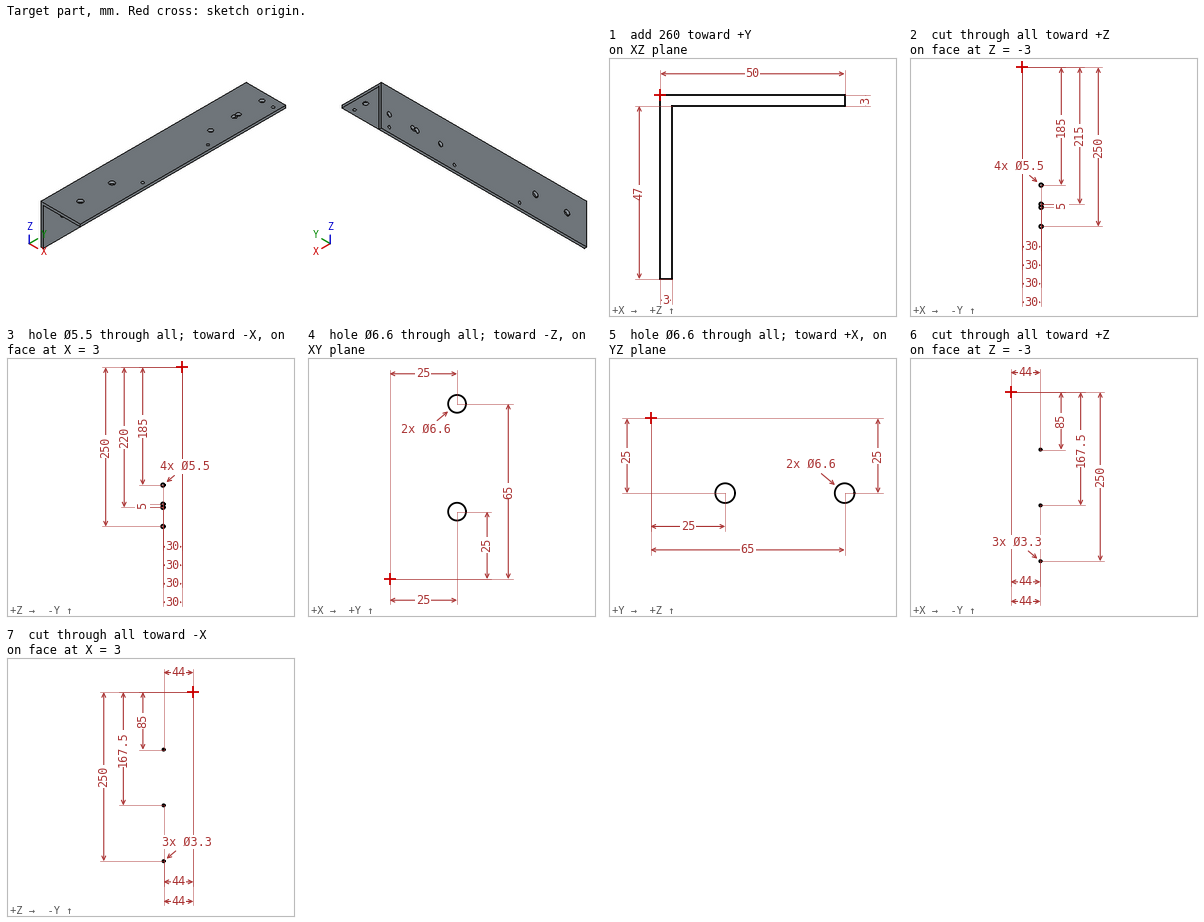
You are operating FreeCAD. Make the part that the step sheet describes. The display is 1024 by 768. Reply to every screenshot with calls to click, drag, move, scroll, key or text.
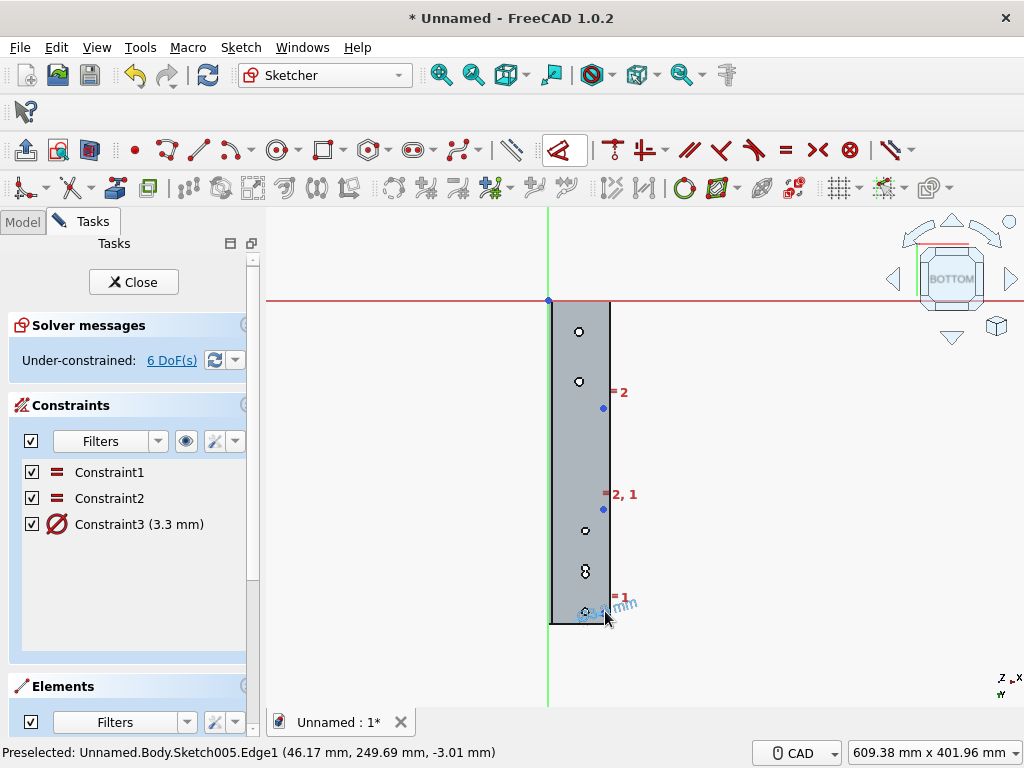
click(603, 613)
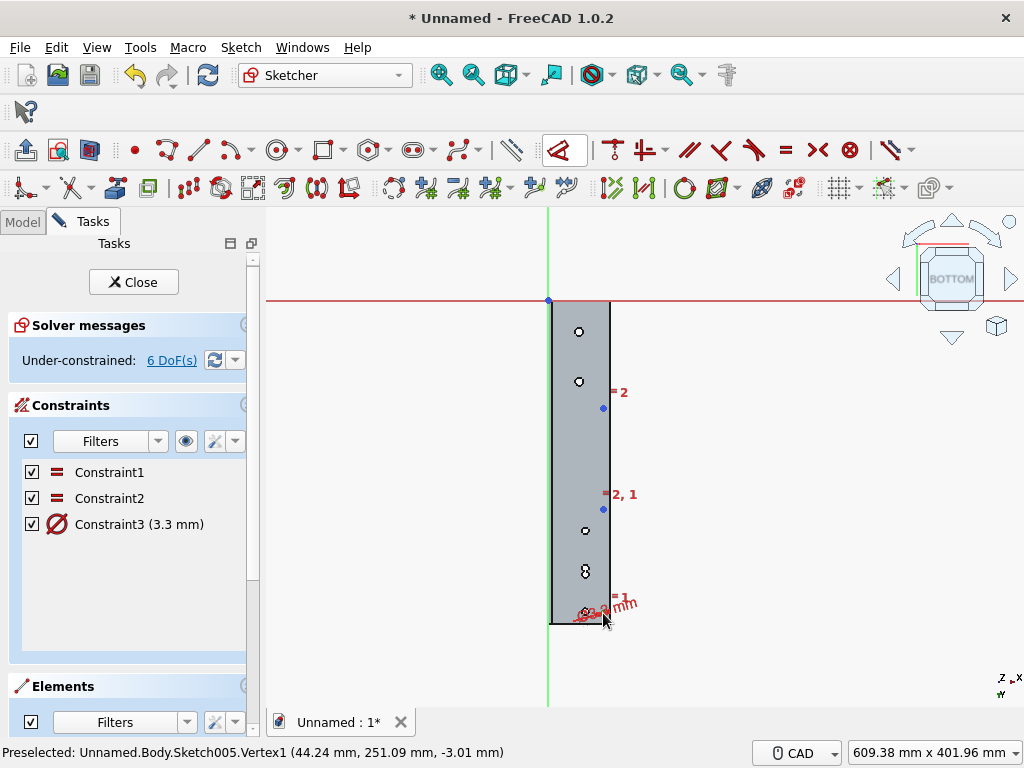
key(l)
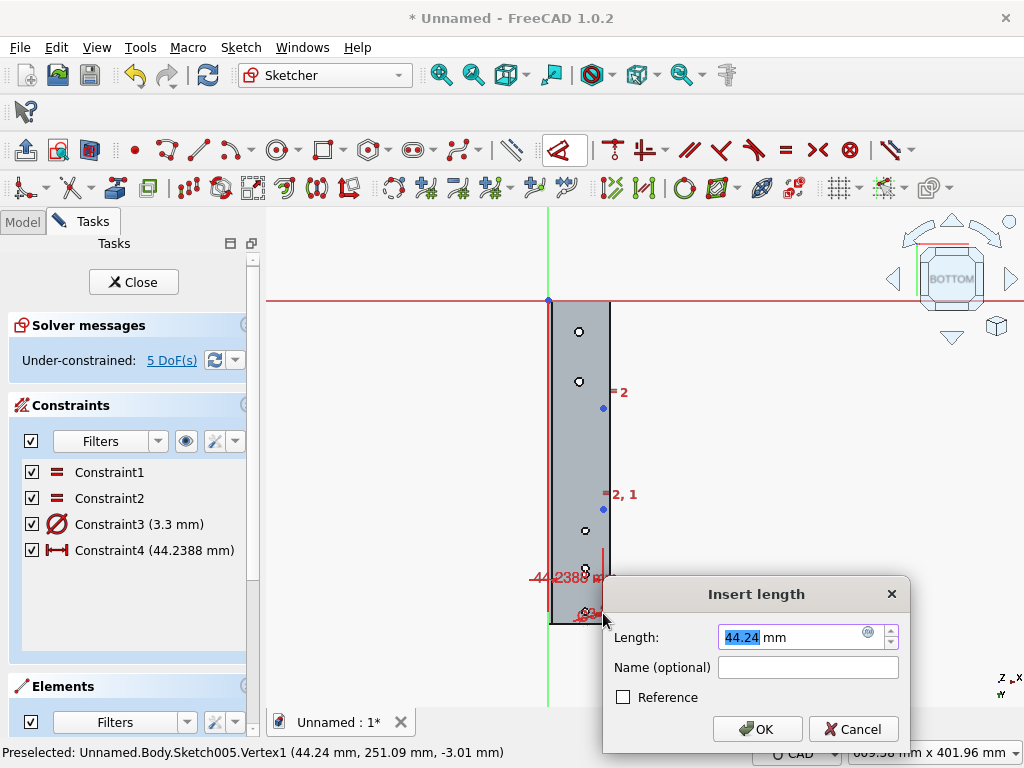
text(44)
key(Return)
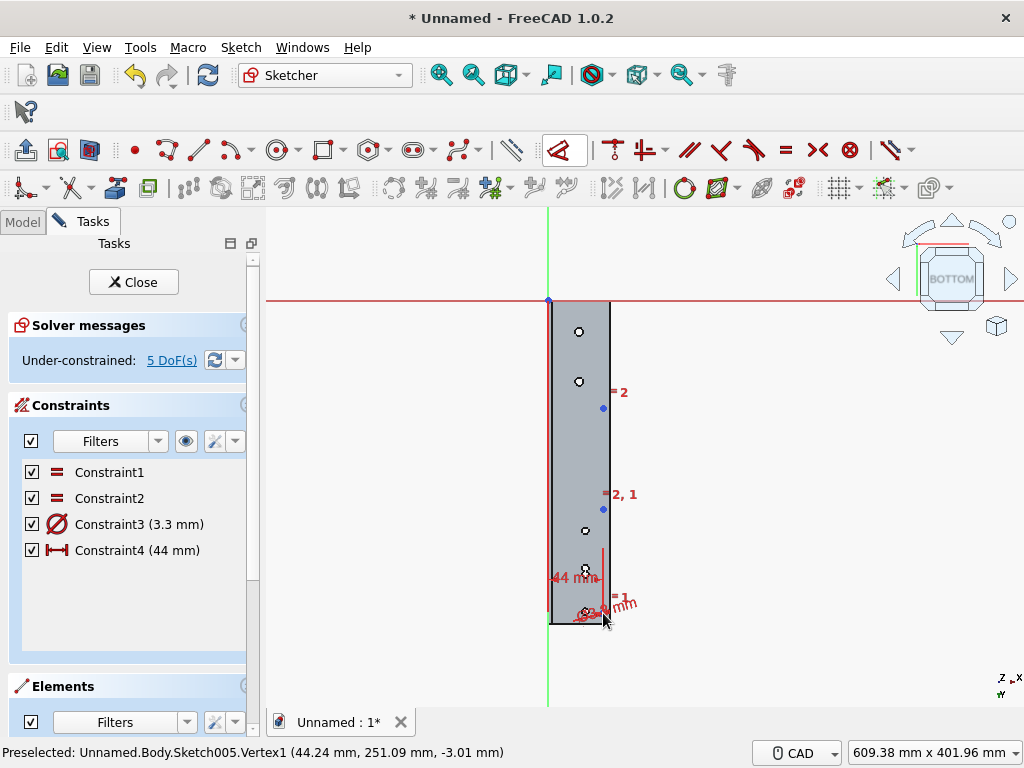
click(603, 510)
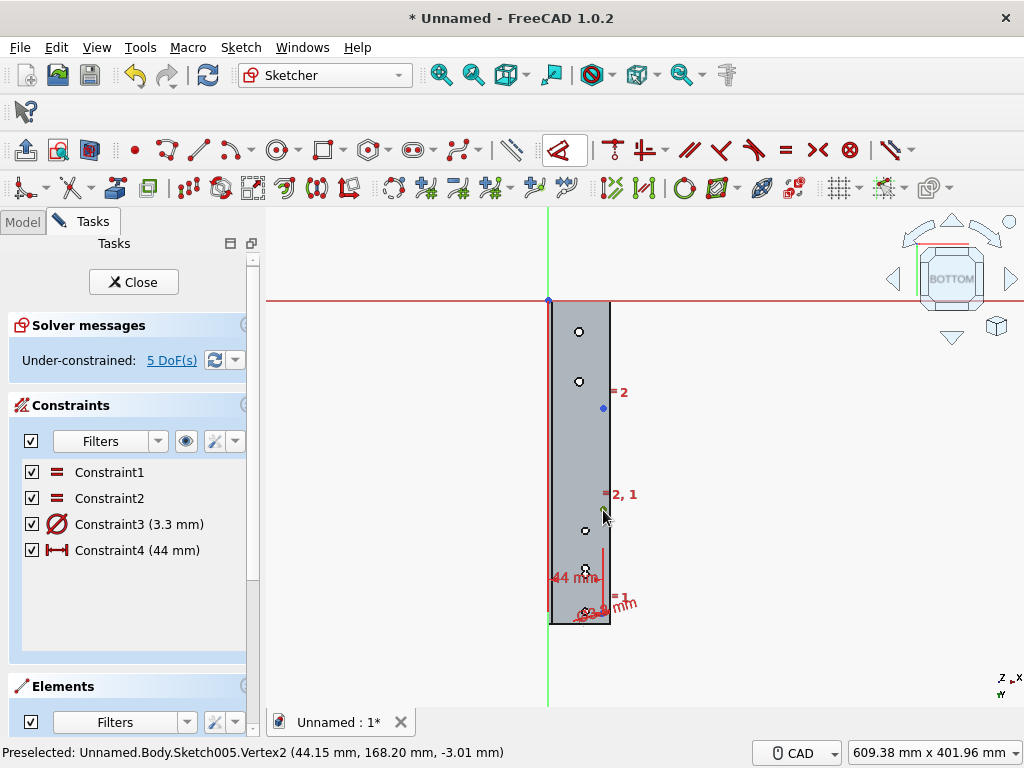
click(582, 150)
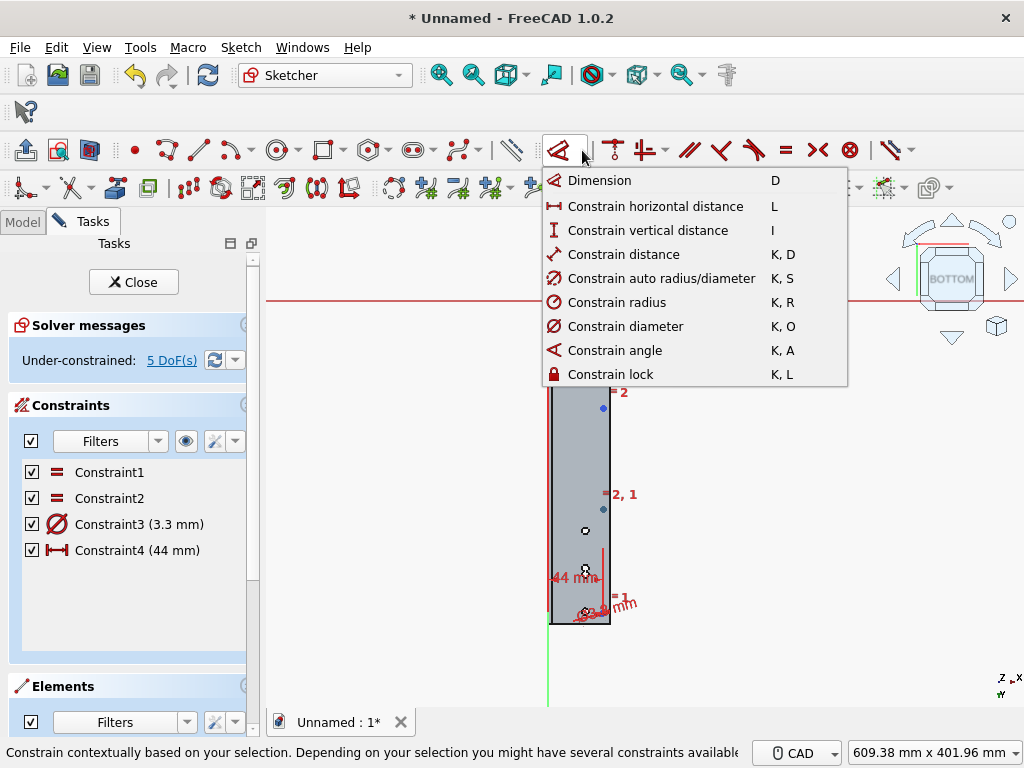
click(695, 206)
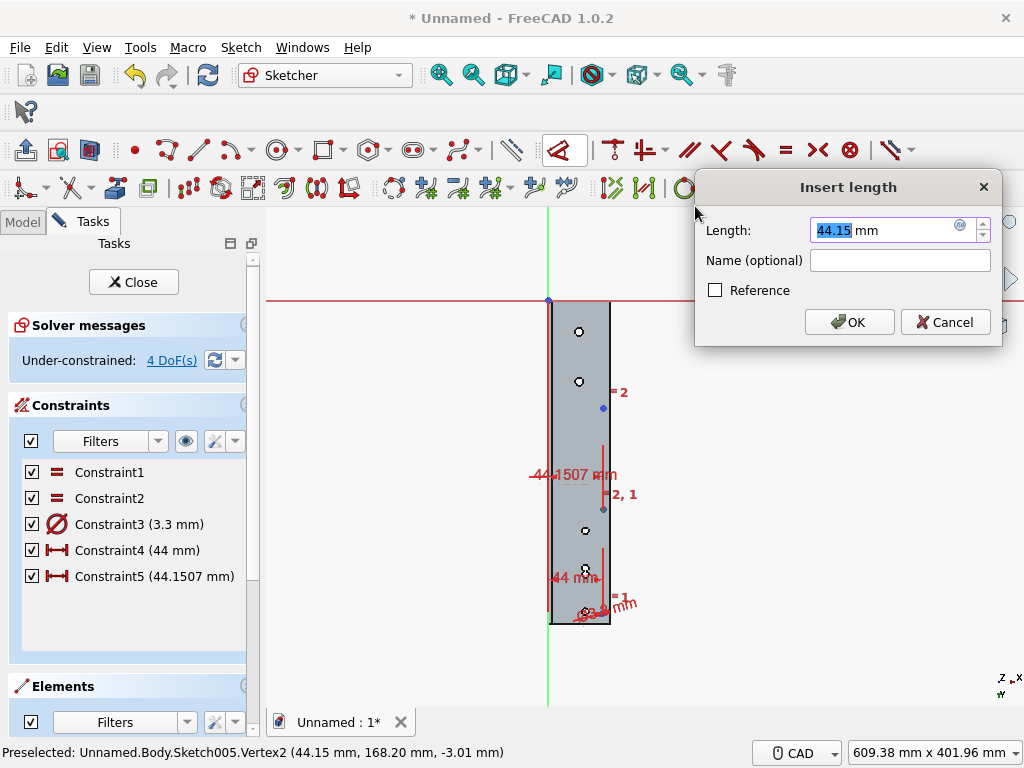
text(44)
key(Return)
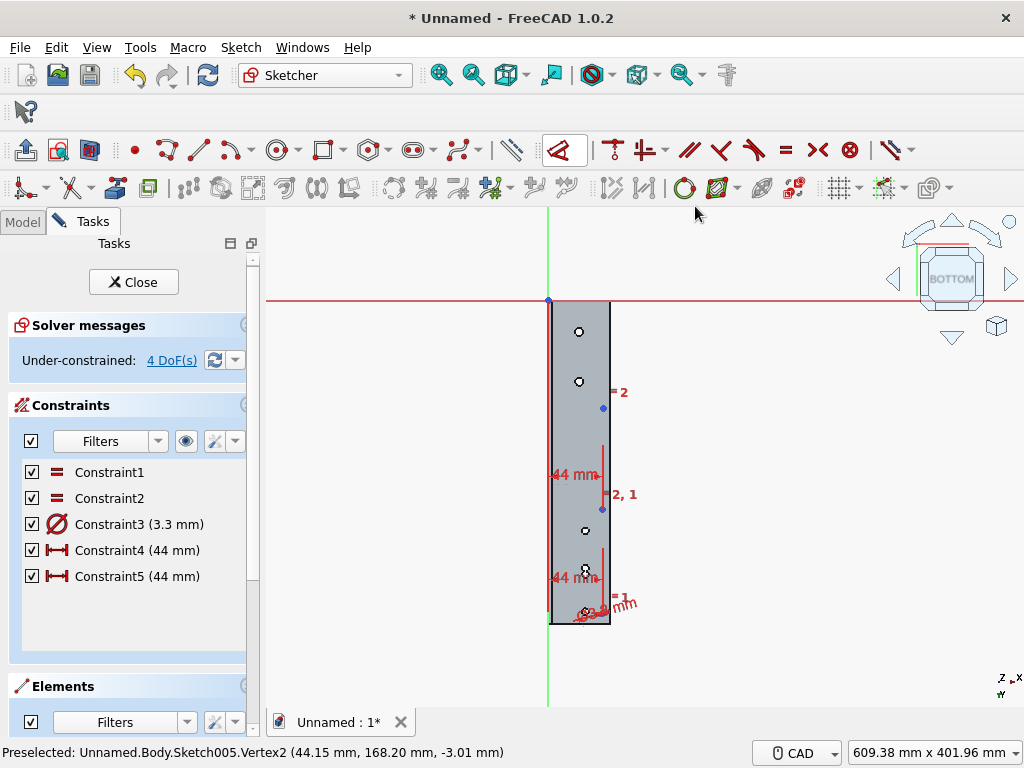
click(603, 408)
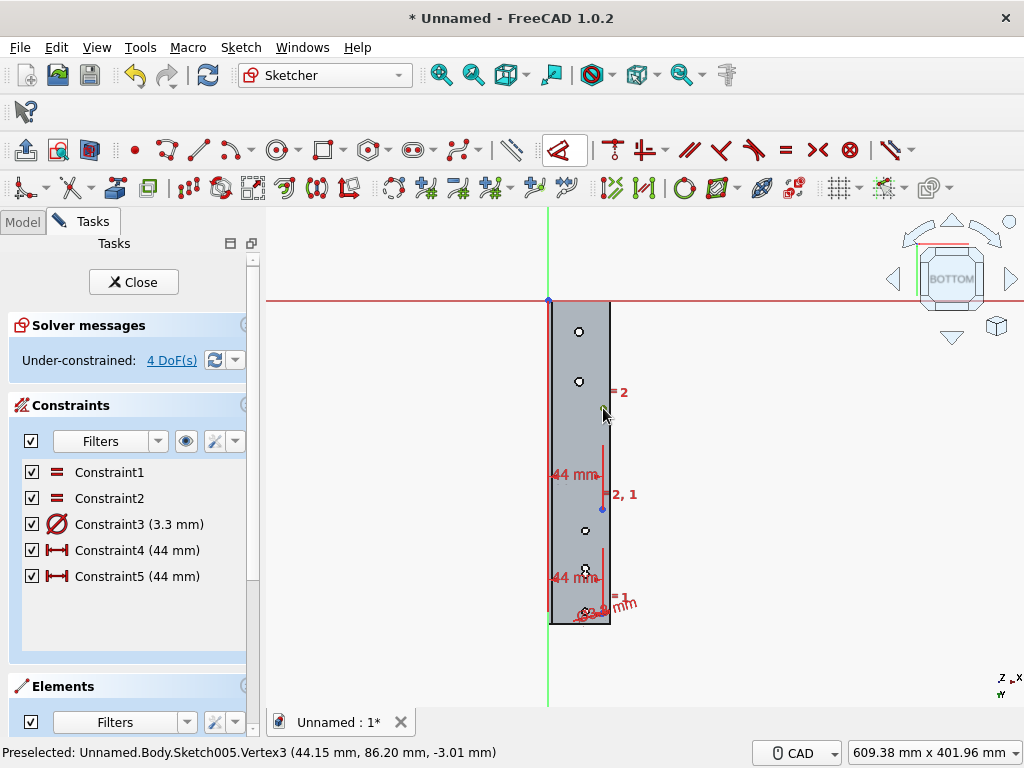
key(l)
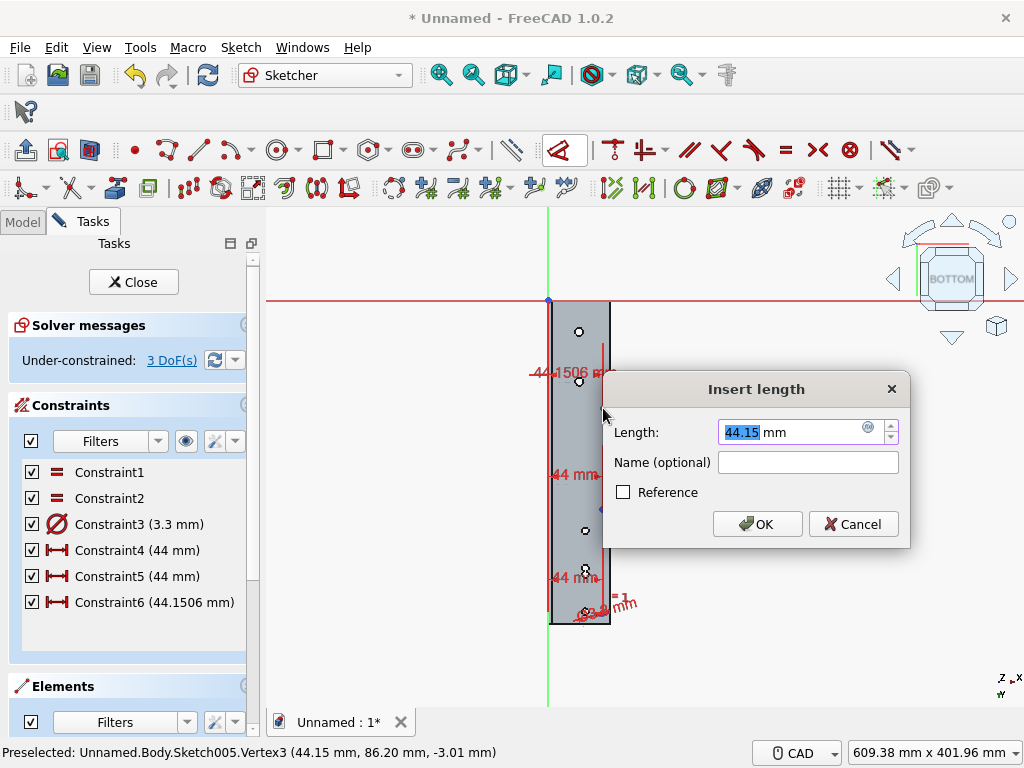
text(44)
key(Return)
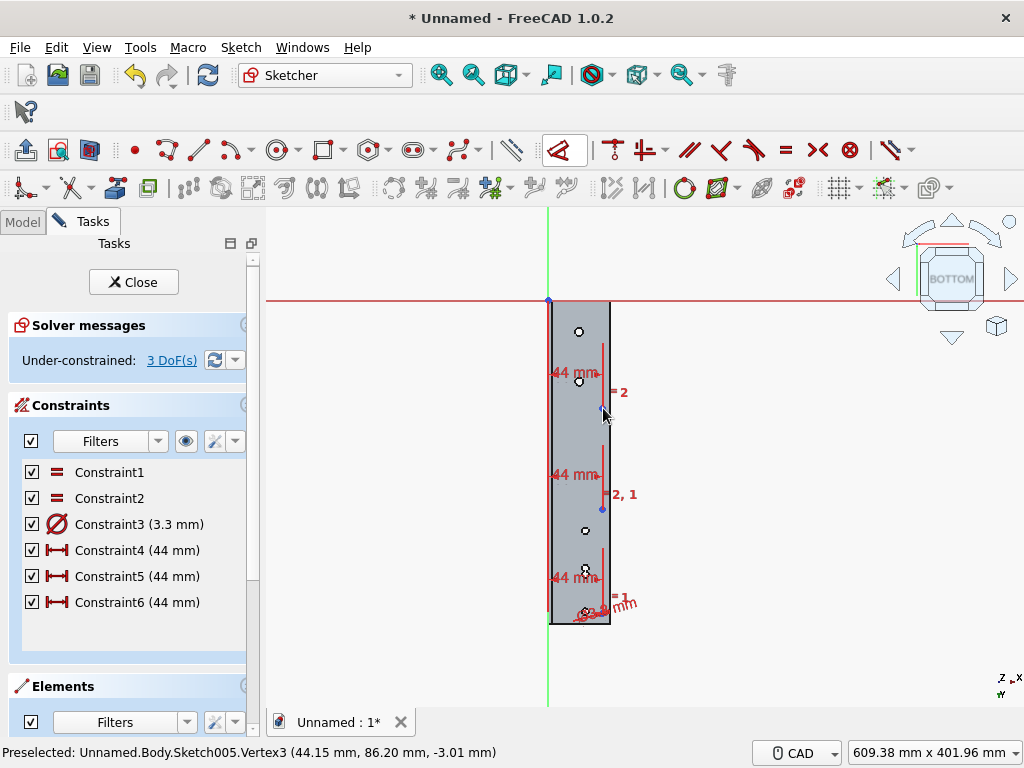
click(603, 408)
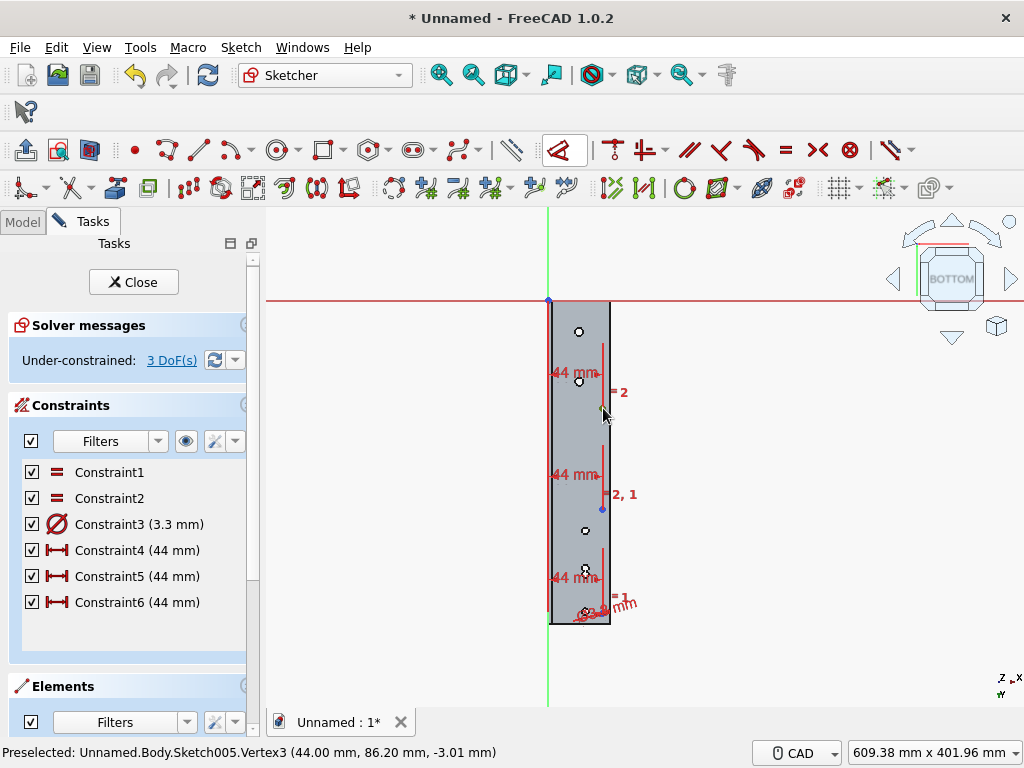
key(i)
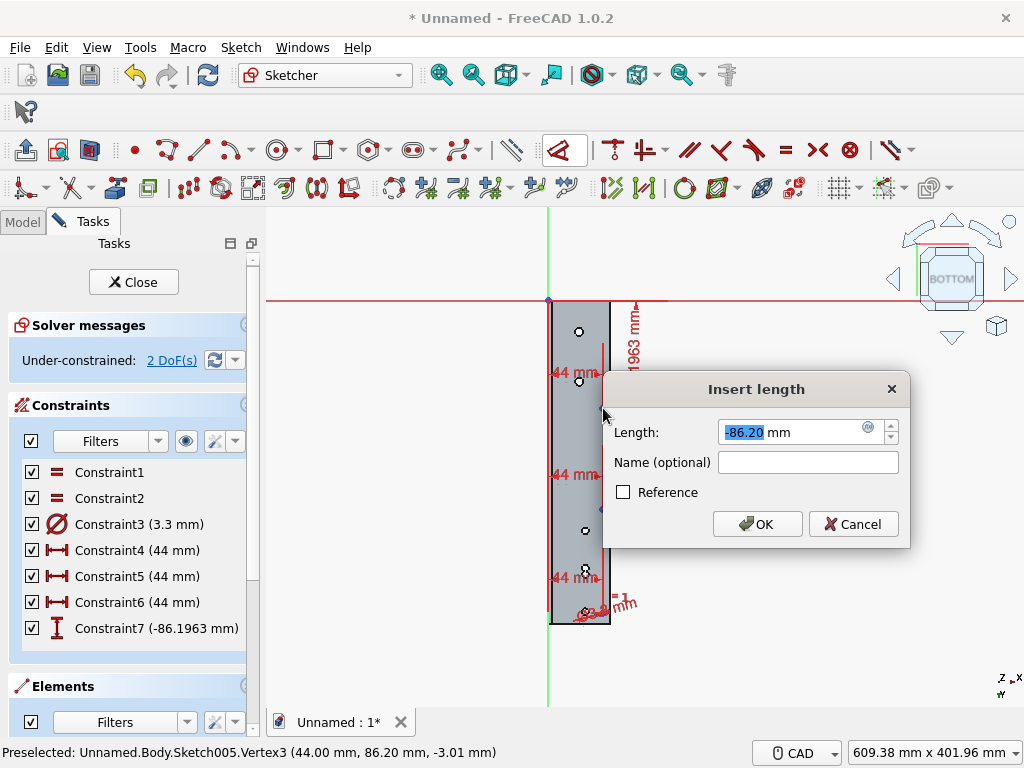
text(-85)
key(Return)